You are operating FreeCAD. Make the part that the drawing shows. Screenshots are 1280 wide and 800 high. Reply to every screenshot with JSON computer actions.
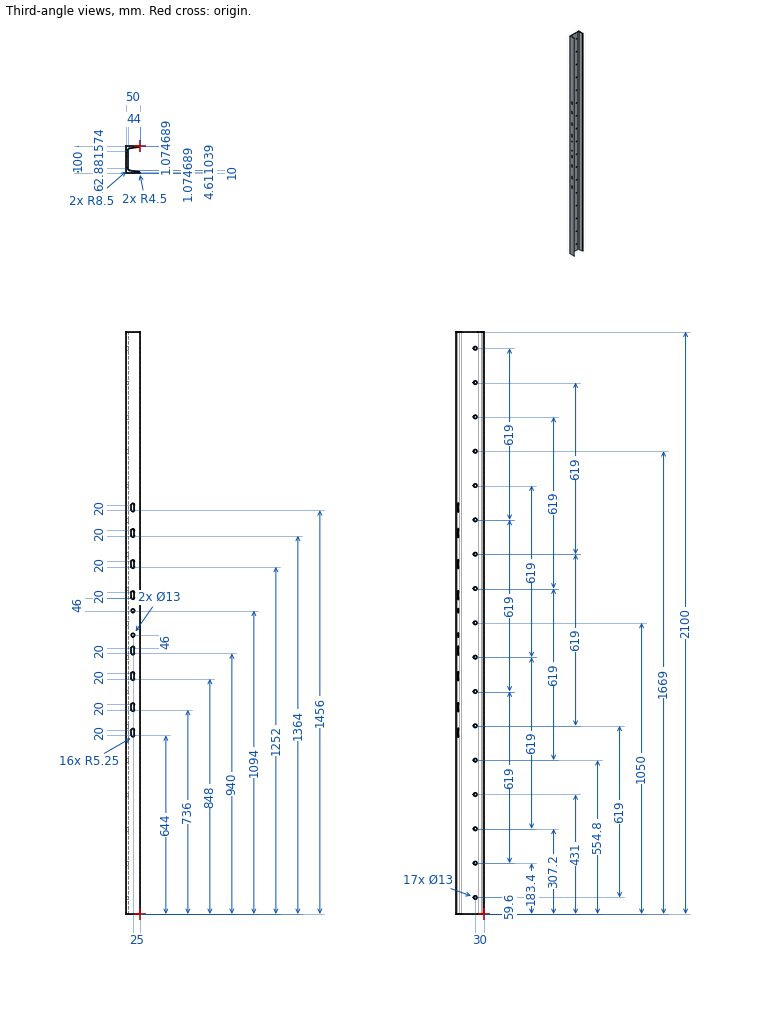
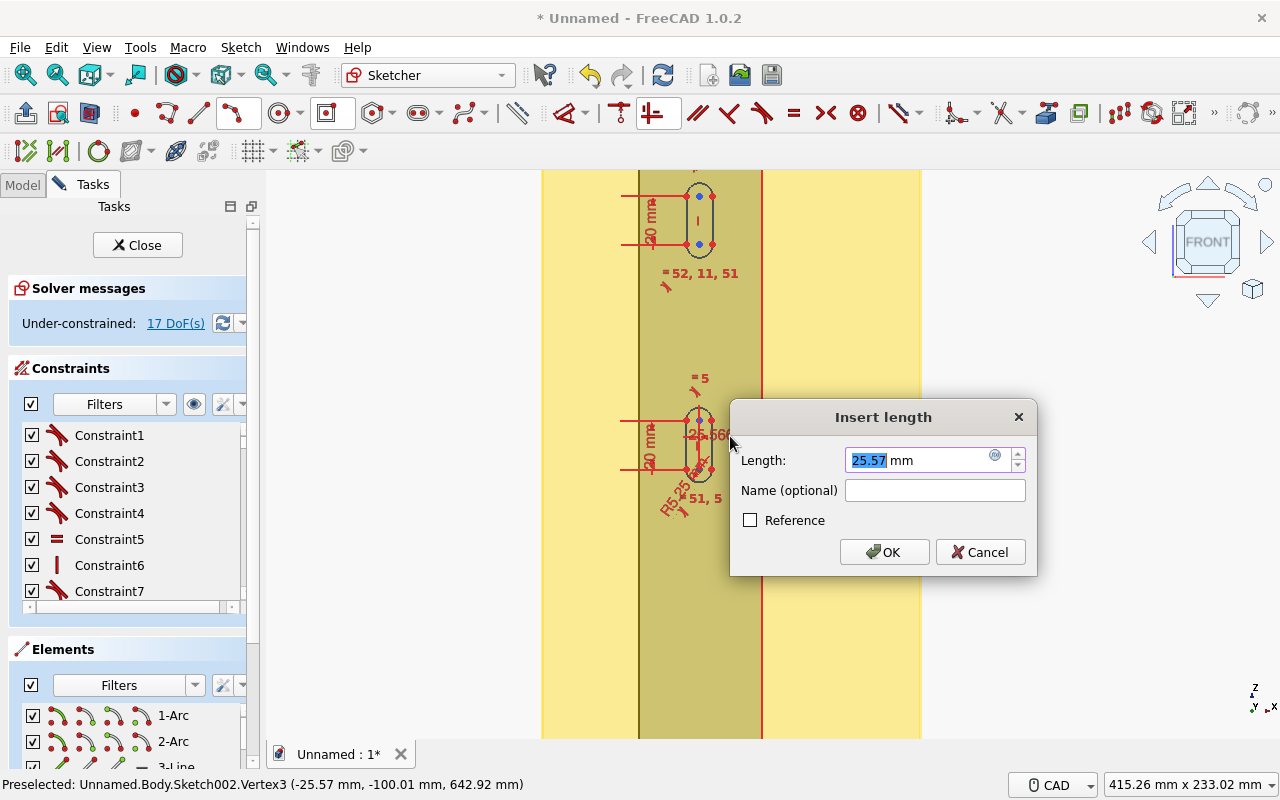
{"action": "type", "text": "25"}
{"action": "key", "text": "Return"}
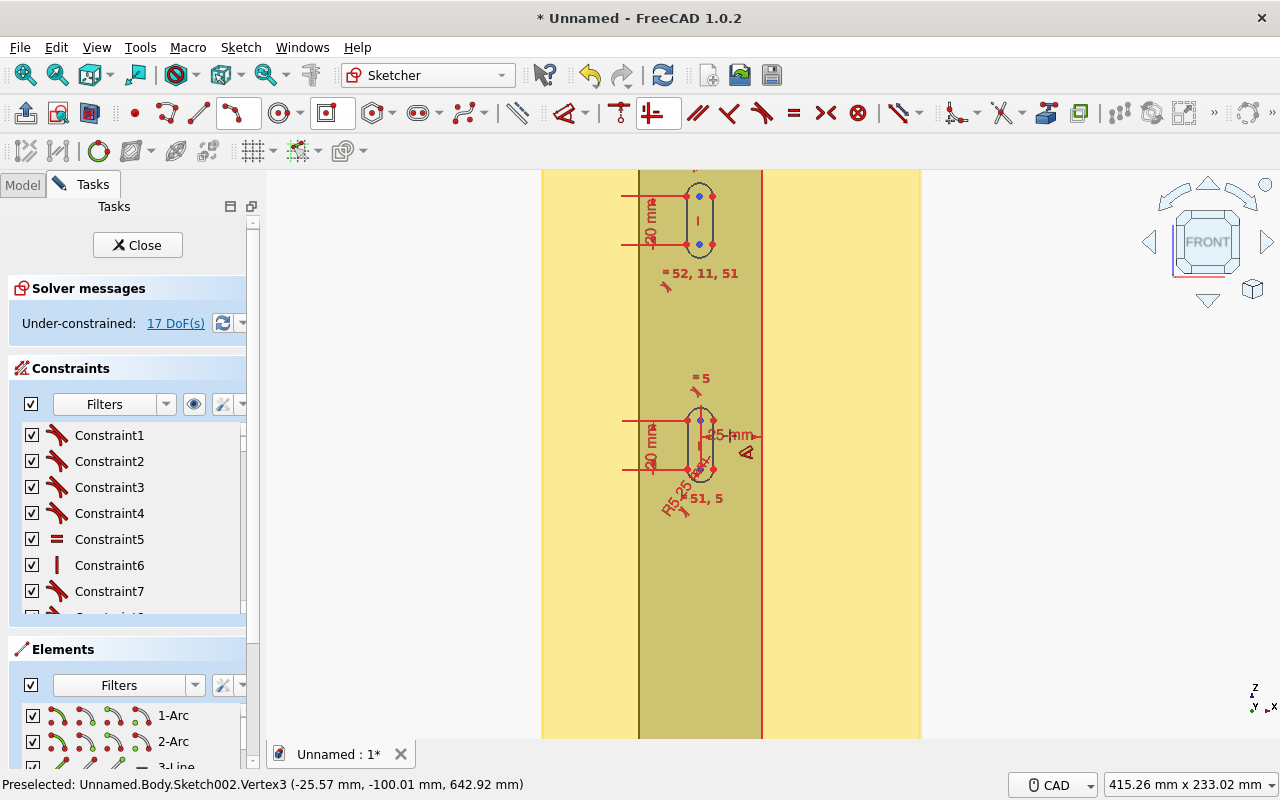
{"action": "left_click", "coordinate": [700, 245]}
{"action": "left_click", "coordinate": [731, 211]}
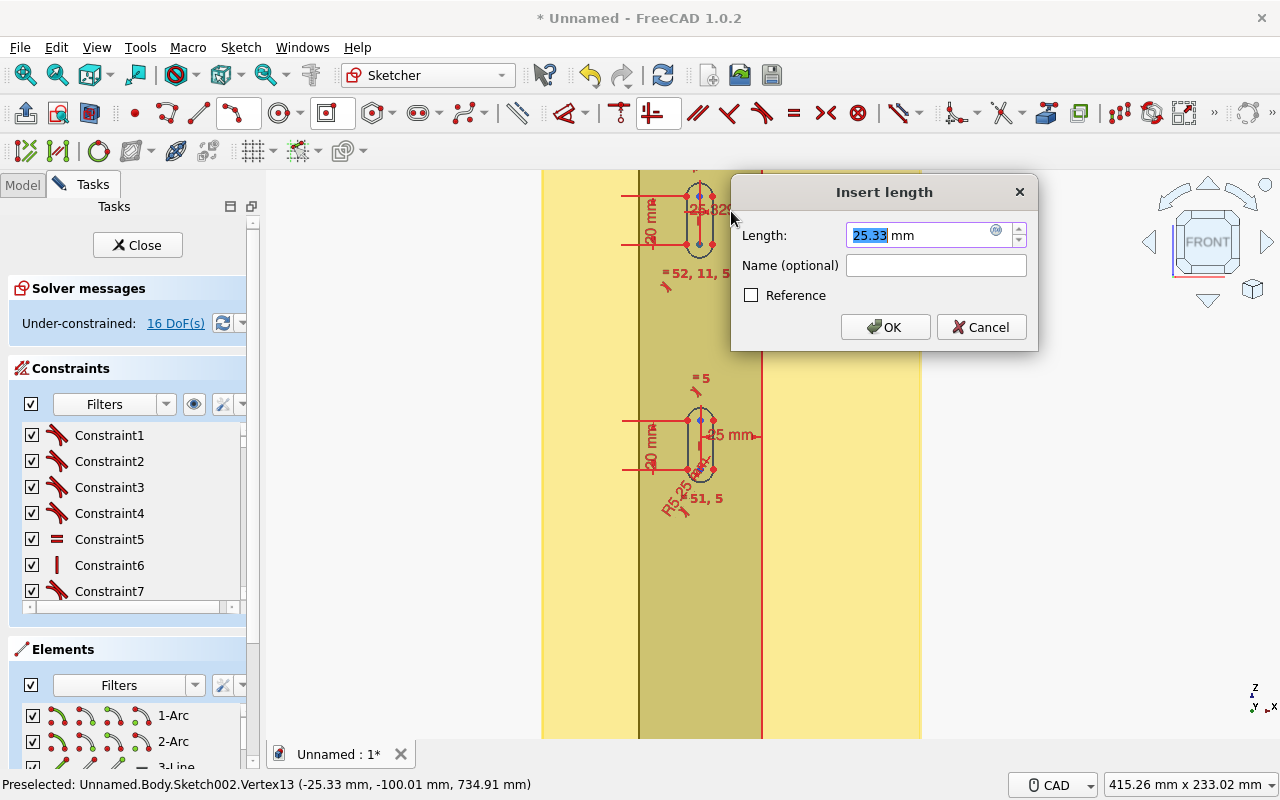
{"action": "type", "text": "25"}
{"action": "key", "text": "Return"}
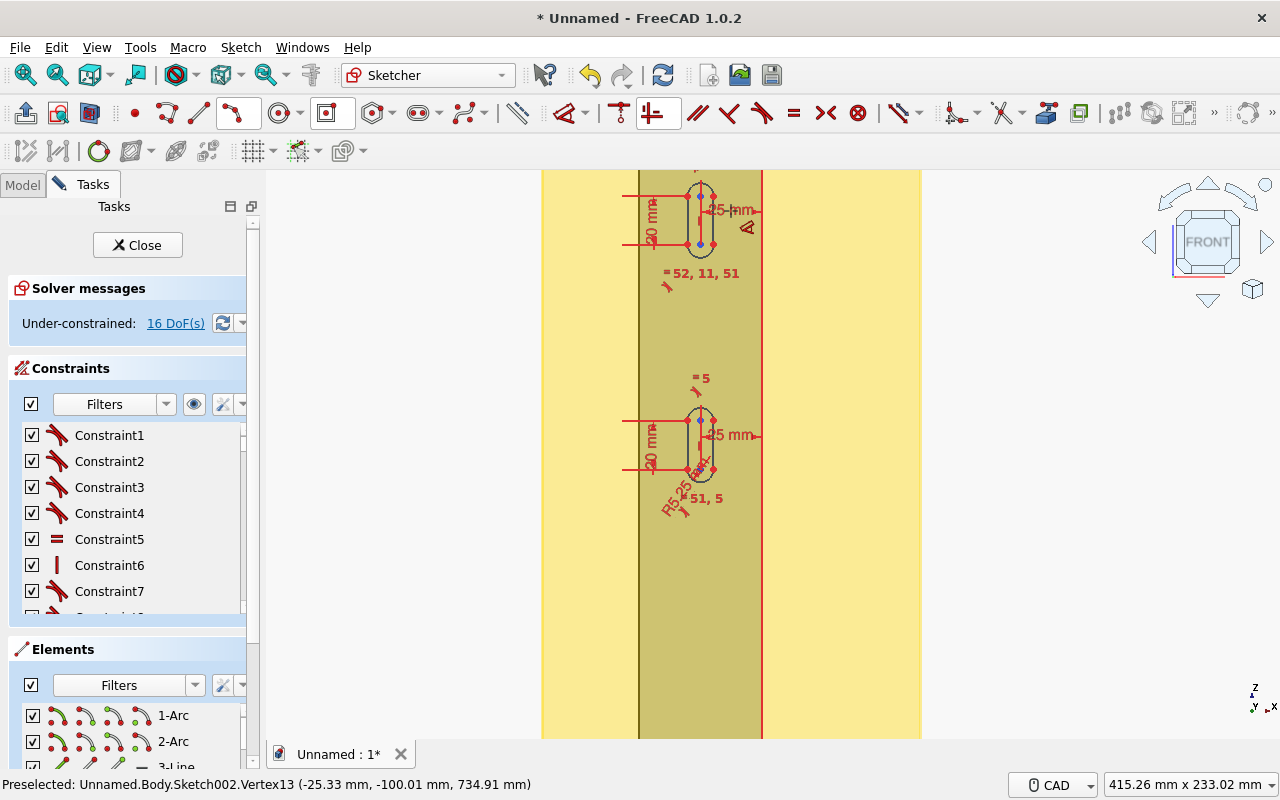
{"action": "scroll", "coordinate": [703, 477], "scroll_direction": "down", "scroll_amount": 12}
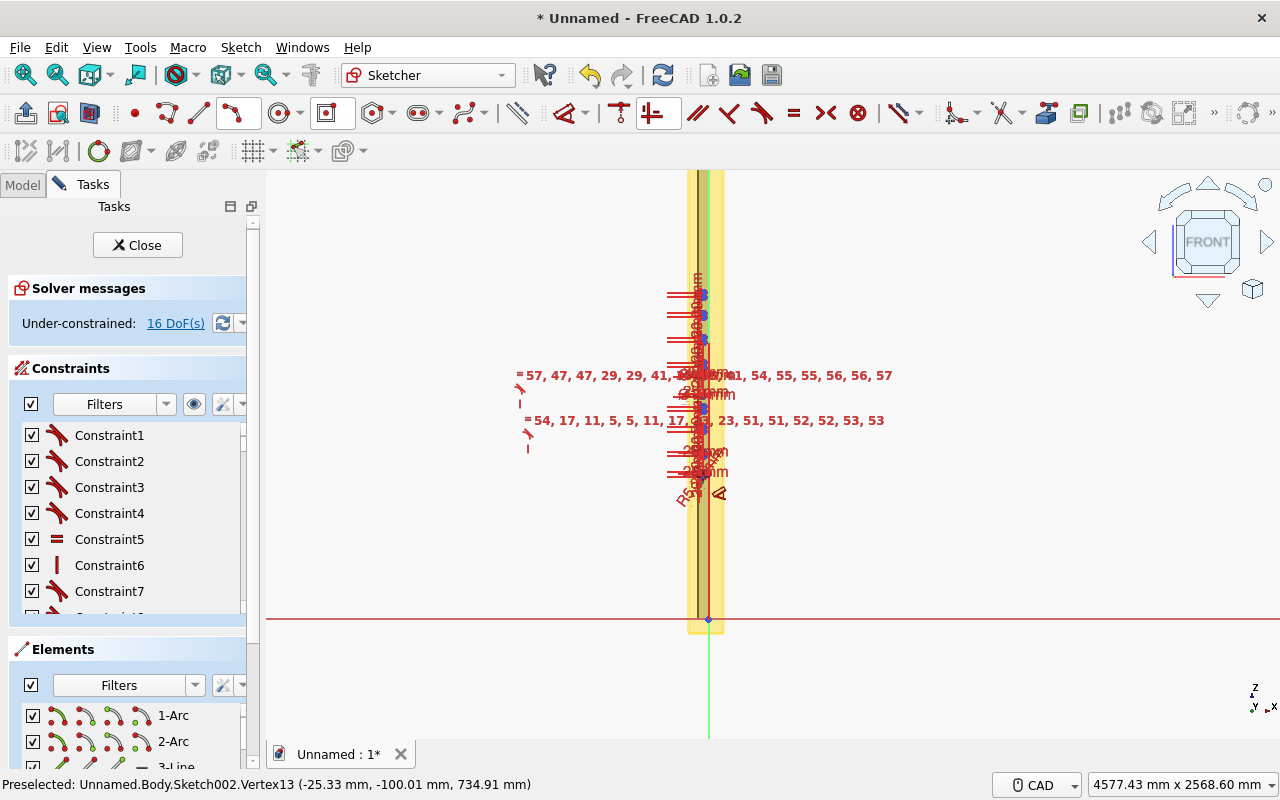
{"action": "scroll", "coordinate": [703, 432], "scroll_direction": "up", "scroll_amount": 12}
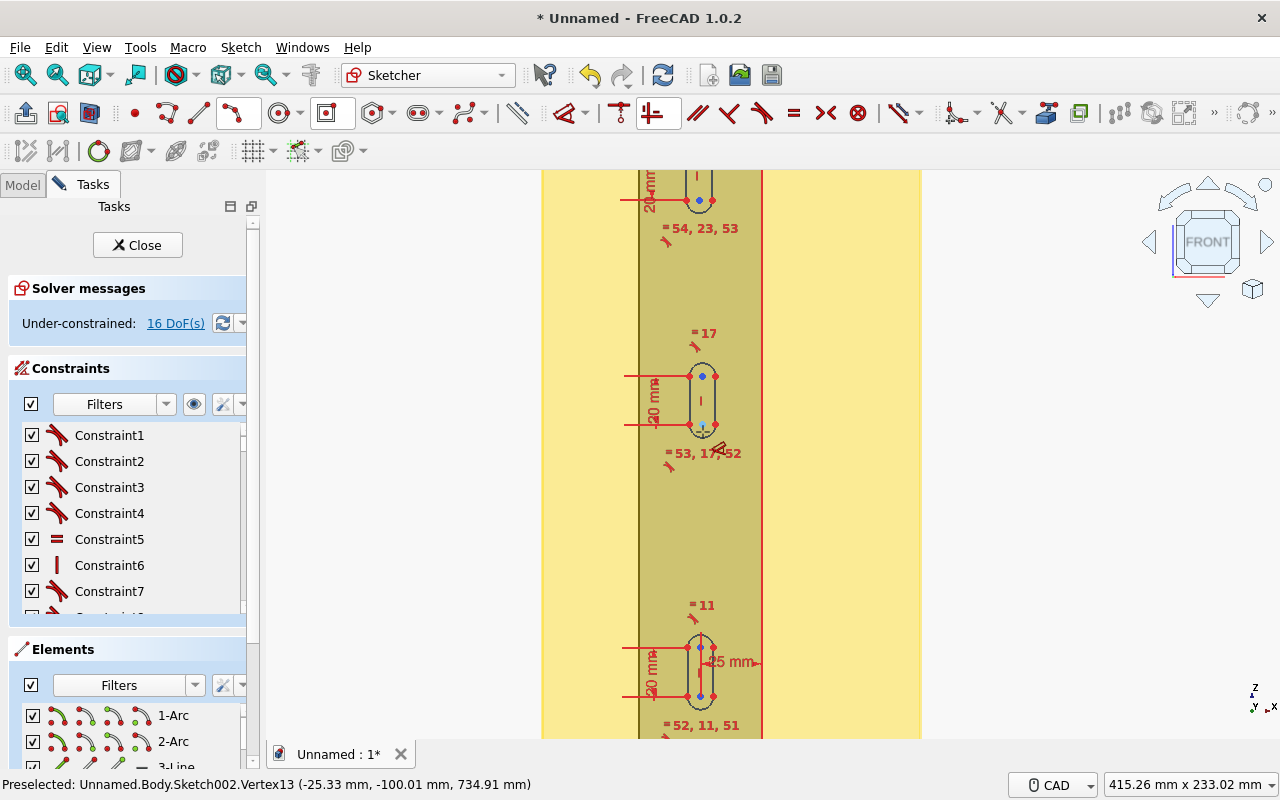
{"action": "left_click", "coordinate": [703, 425]}
{"action": "left_click", "coordinate": [732, 391]}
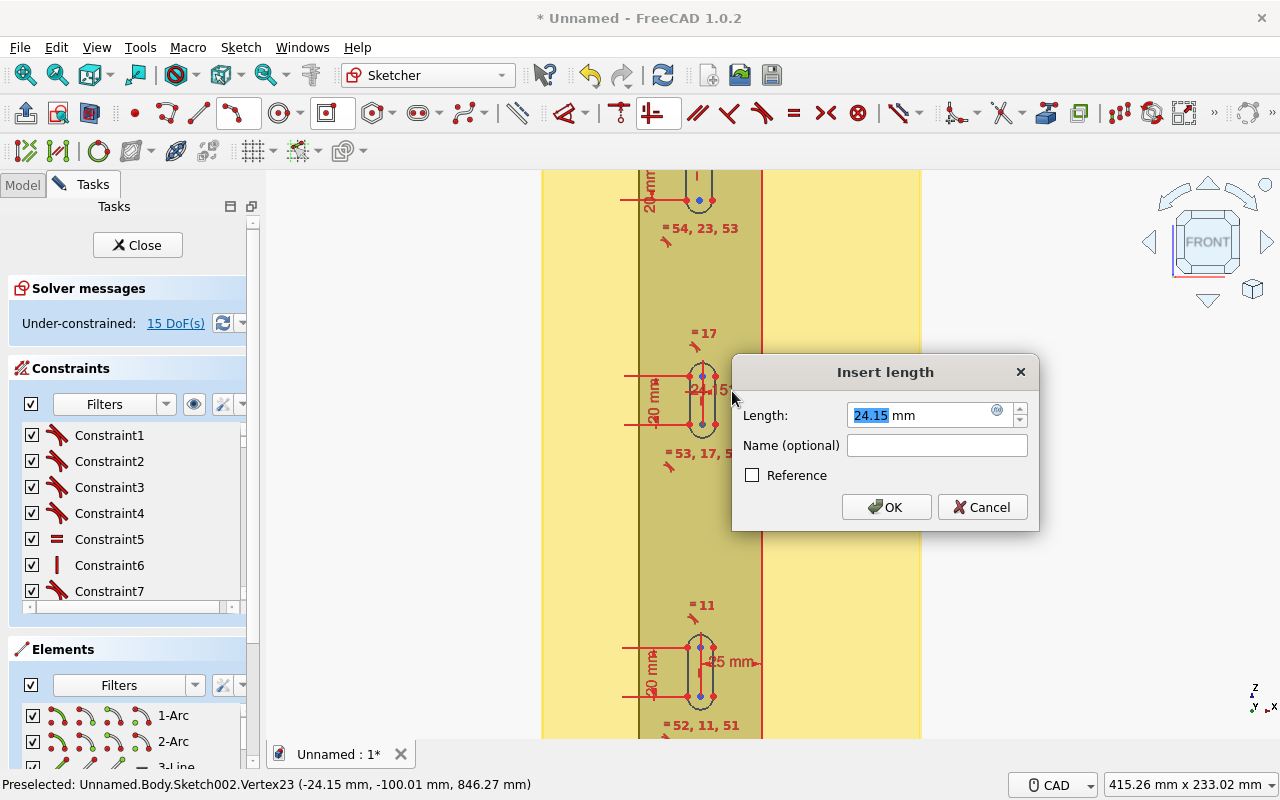
{"action": "type", "text": "25"}
{"action": "key", "text": "Return"}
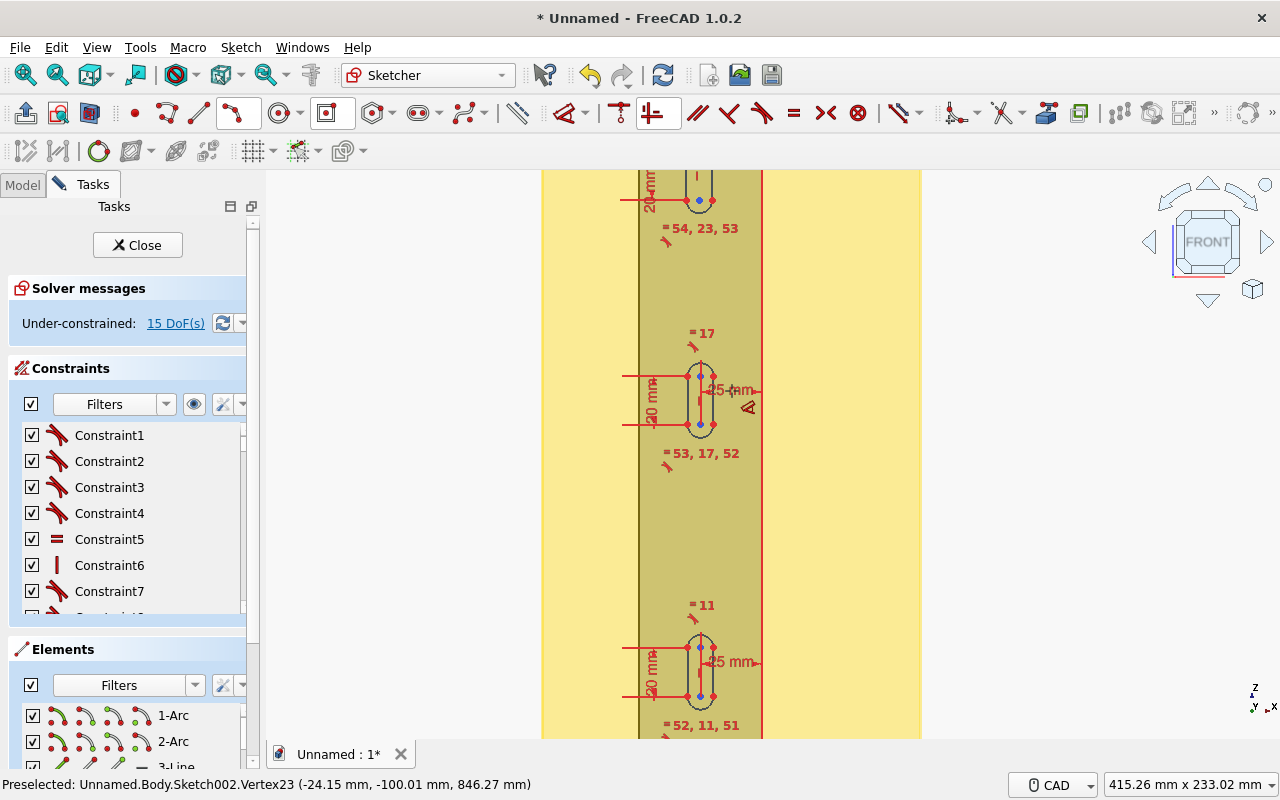
{"action": "left_click", "coordinate": [699, 200]}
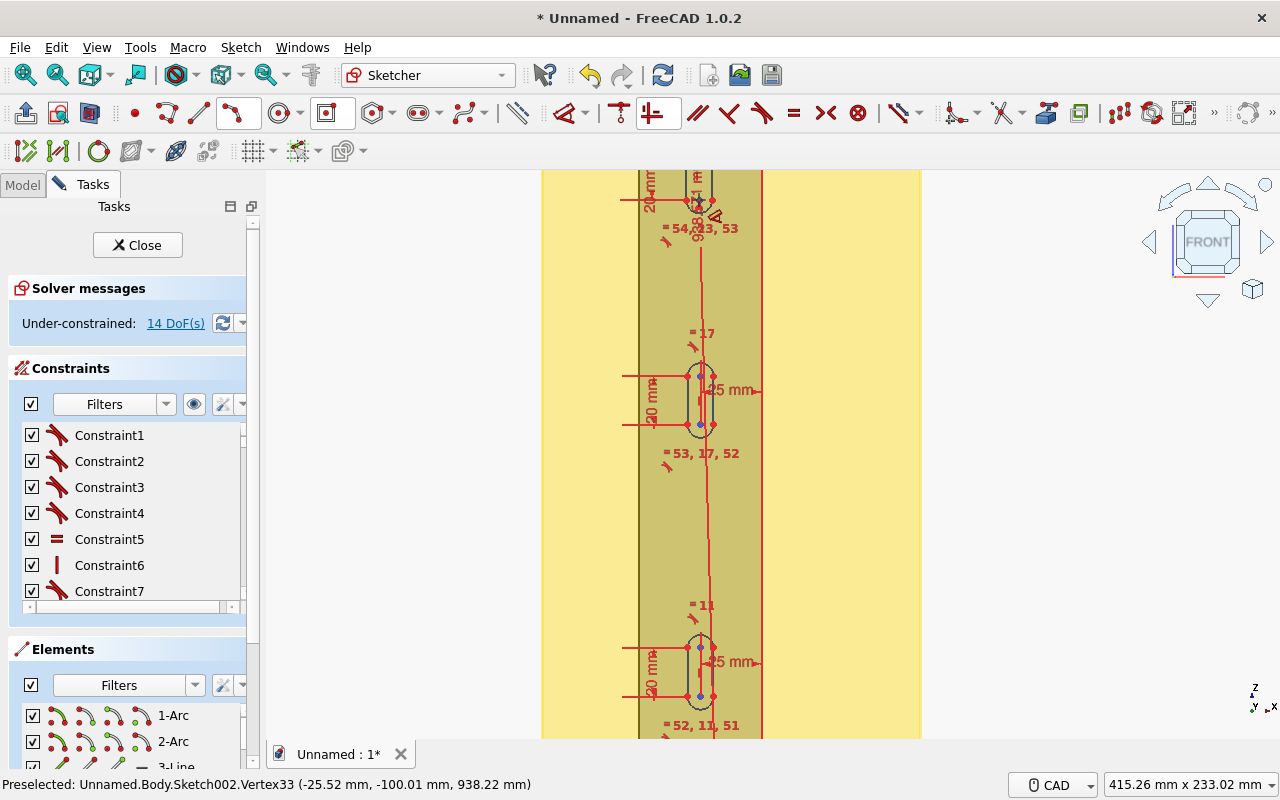
{"action": "key", "text": "Escape"}
{"action": "key", "text": "Escape"}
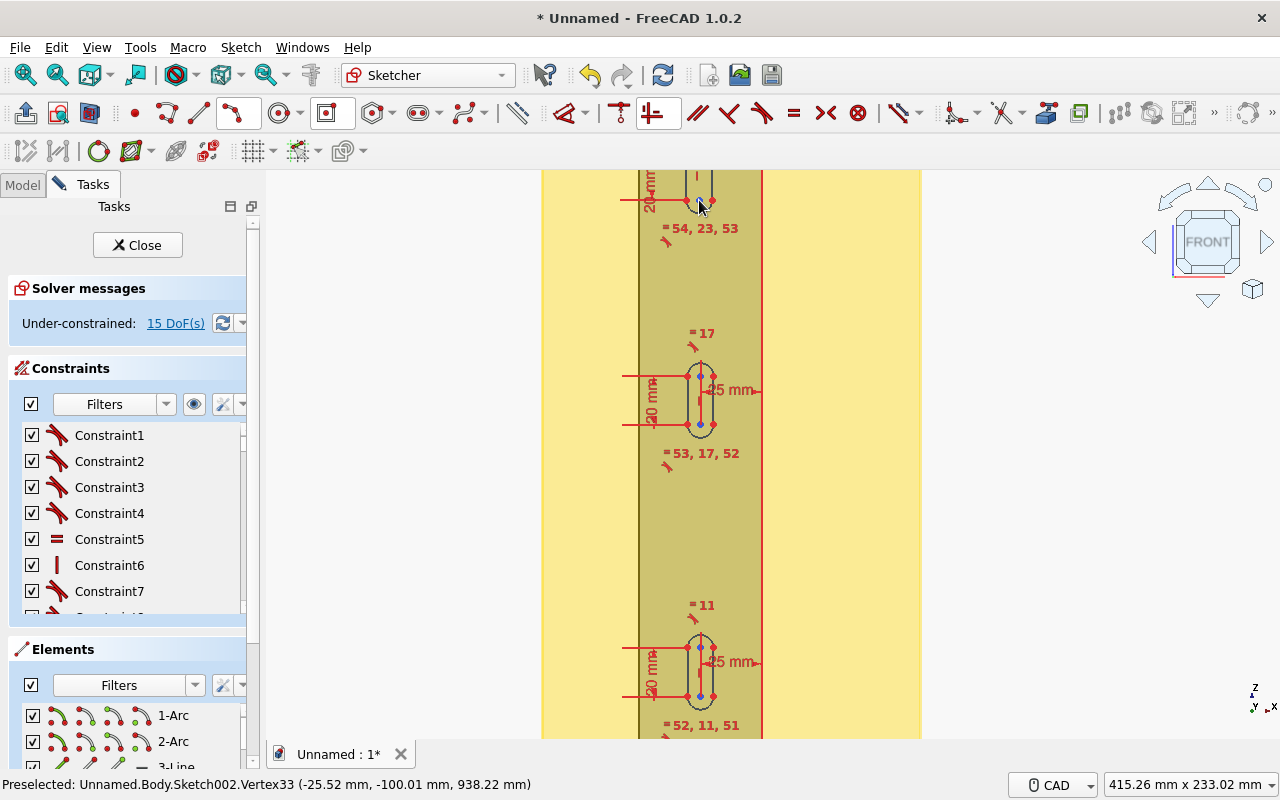
{"action": "left_click", "coordinate": [699, 200]}